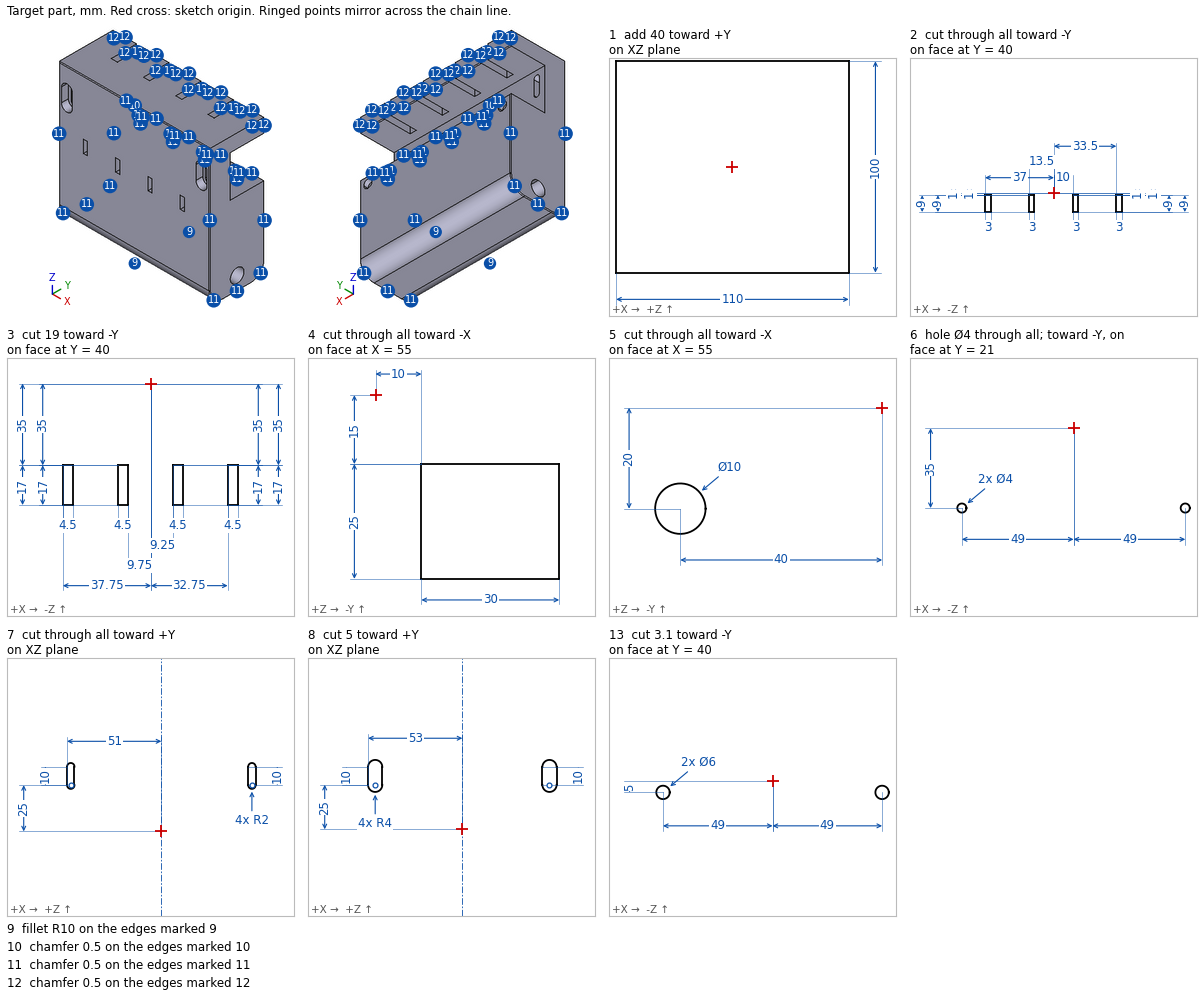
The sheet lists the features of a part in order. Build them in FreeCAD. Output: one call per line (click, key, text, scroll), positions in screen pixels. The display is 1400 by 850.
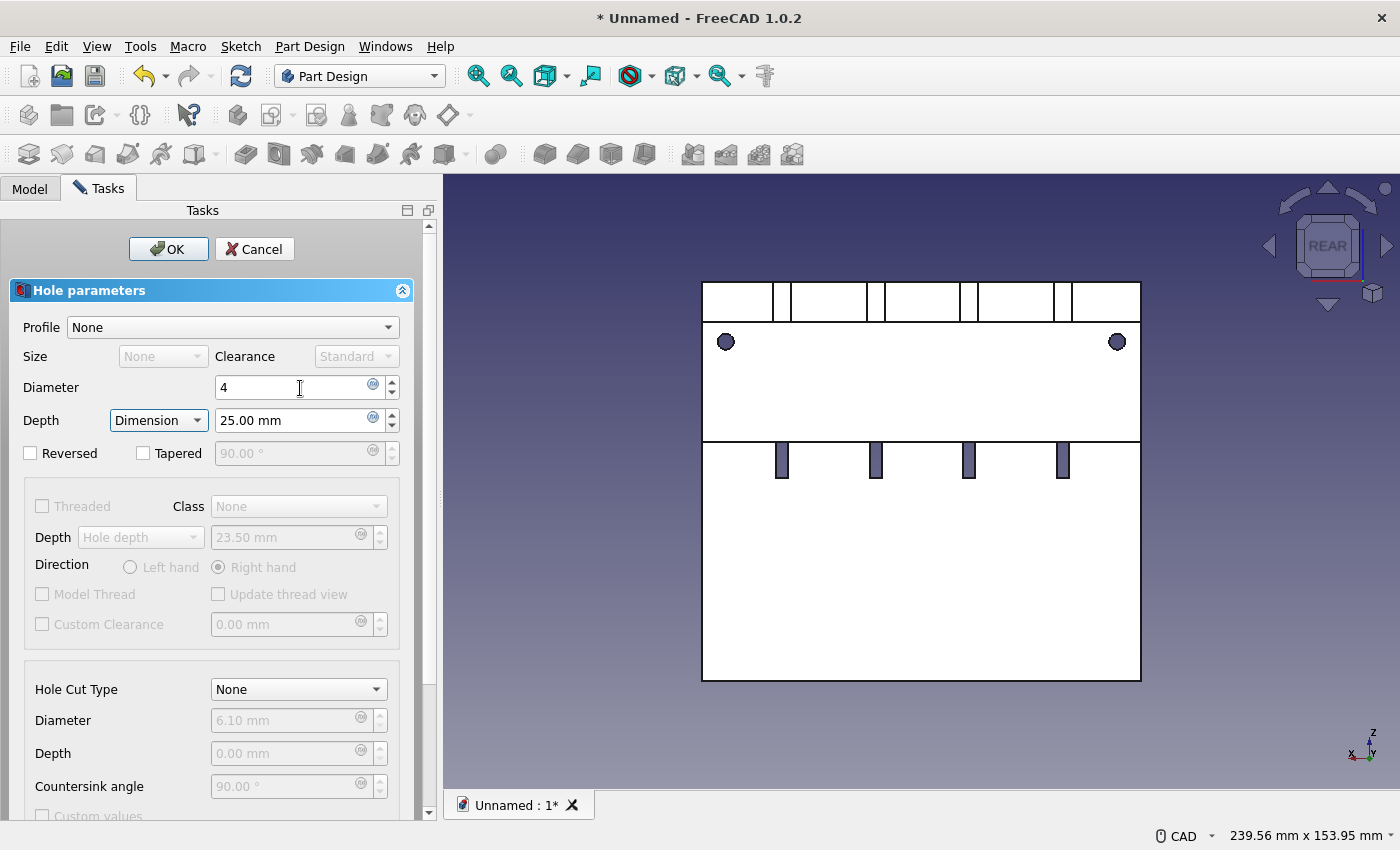
click(160, 420)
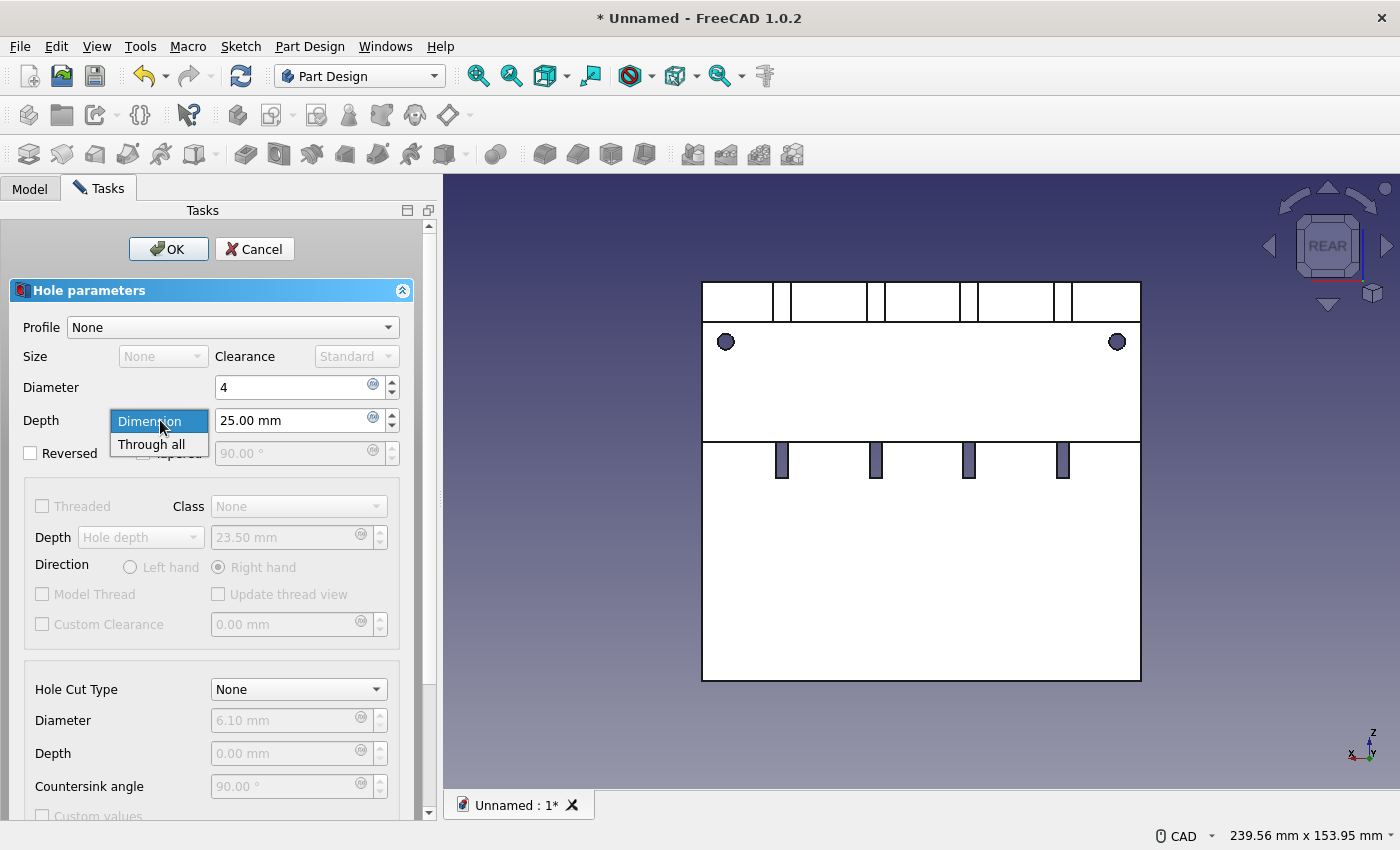
click(158, 444)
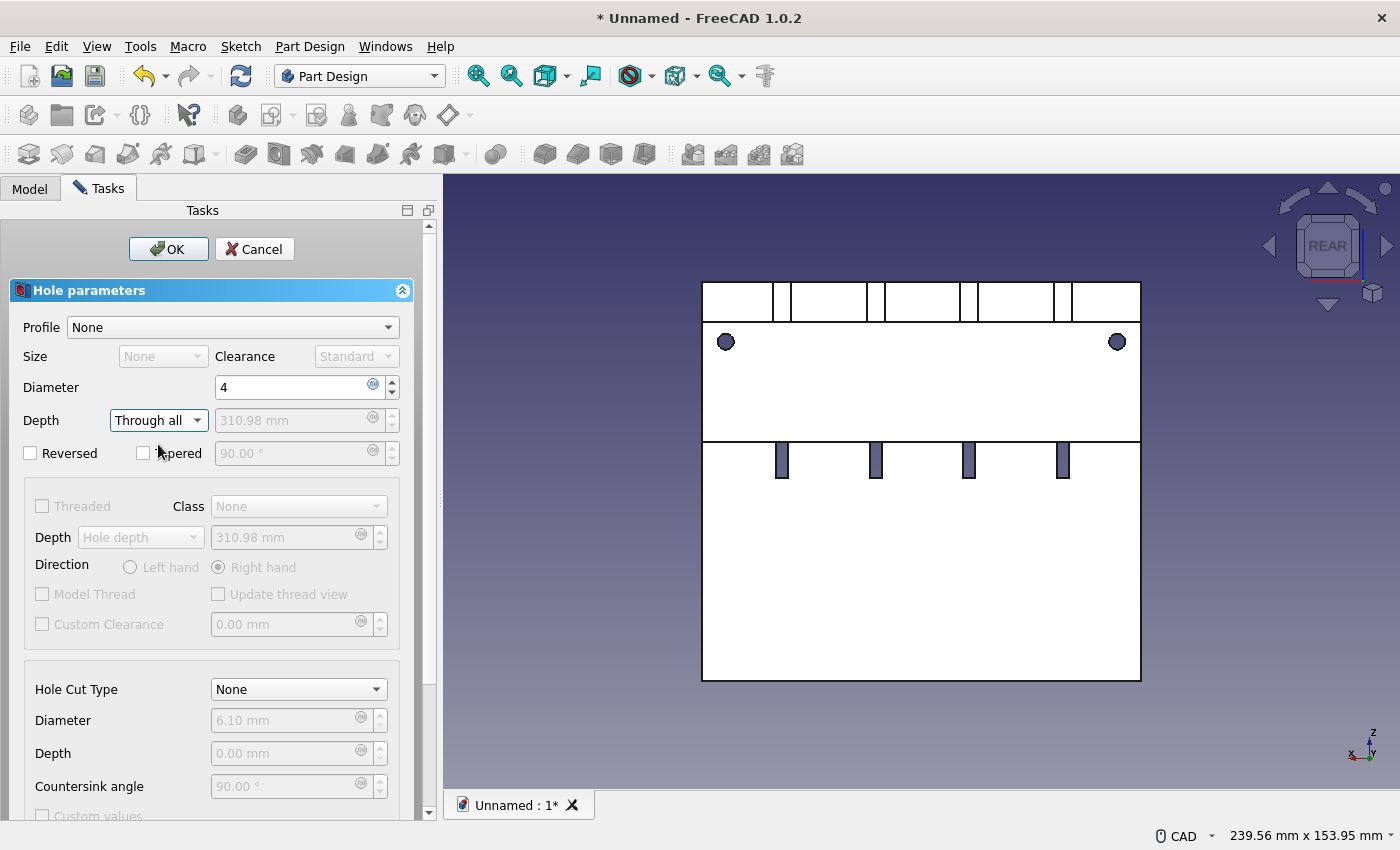
click(169, 249)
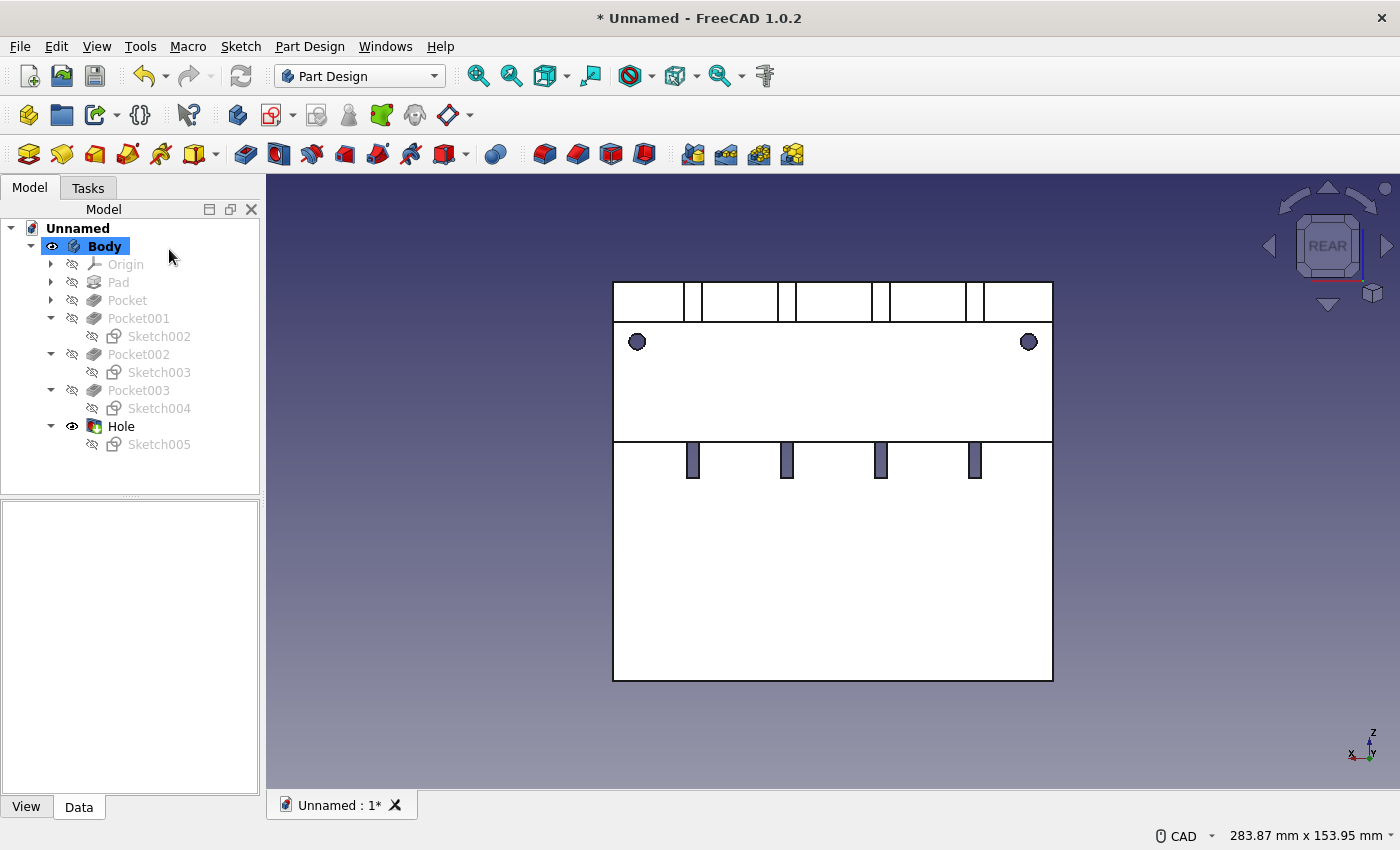
click(270, 116)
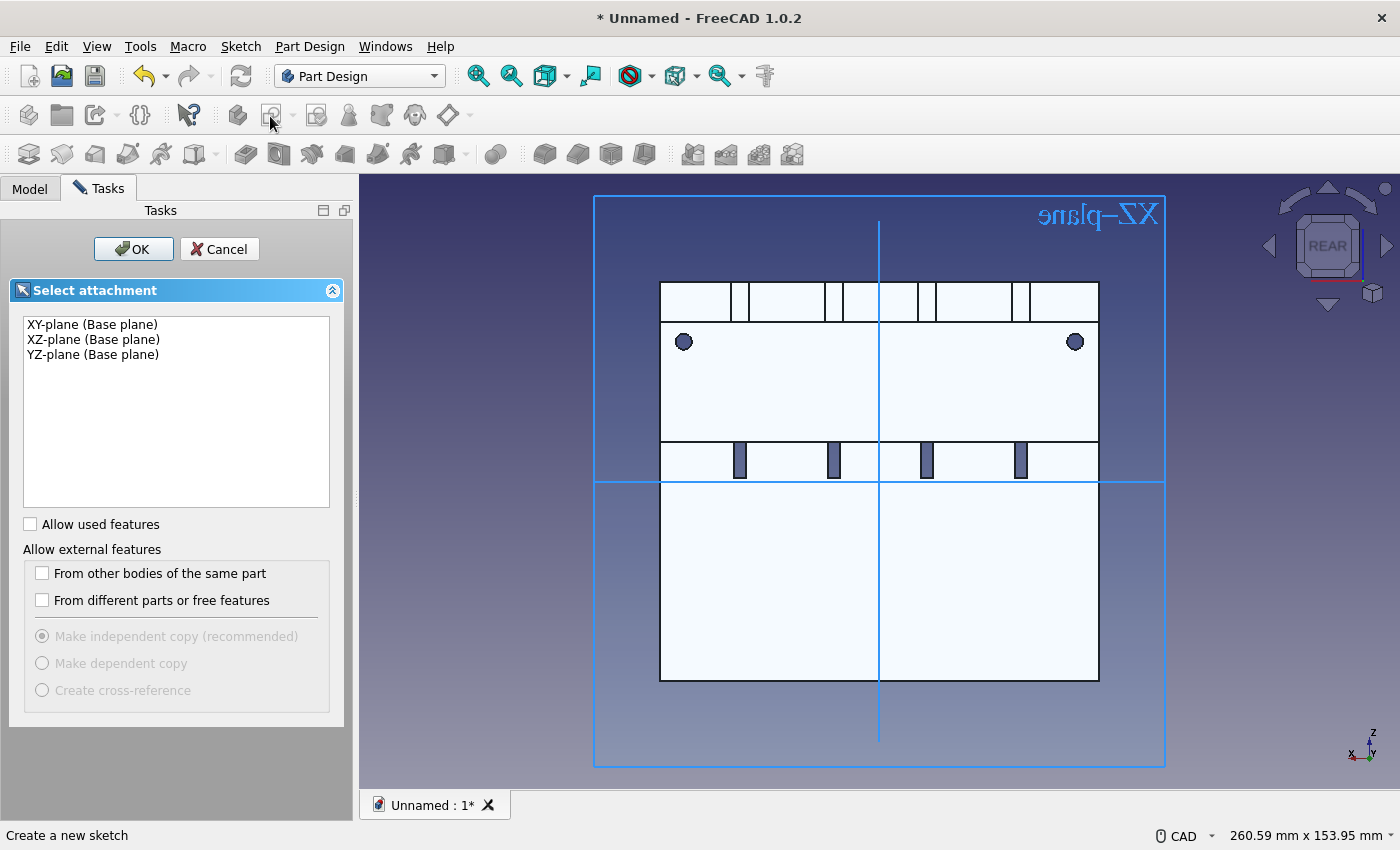
click(84, 340)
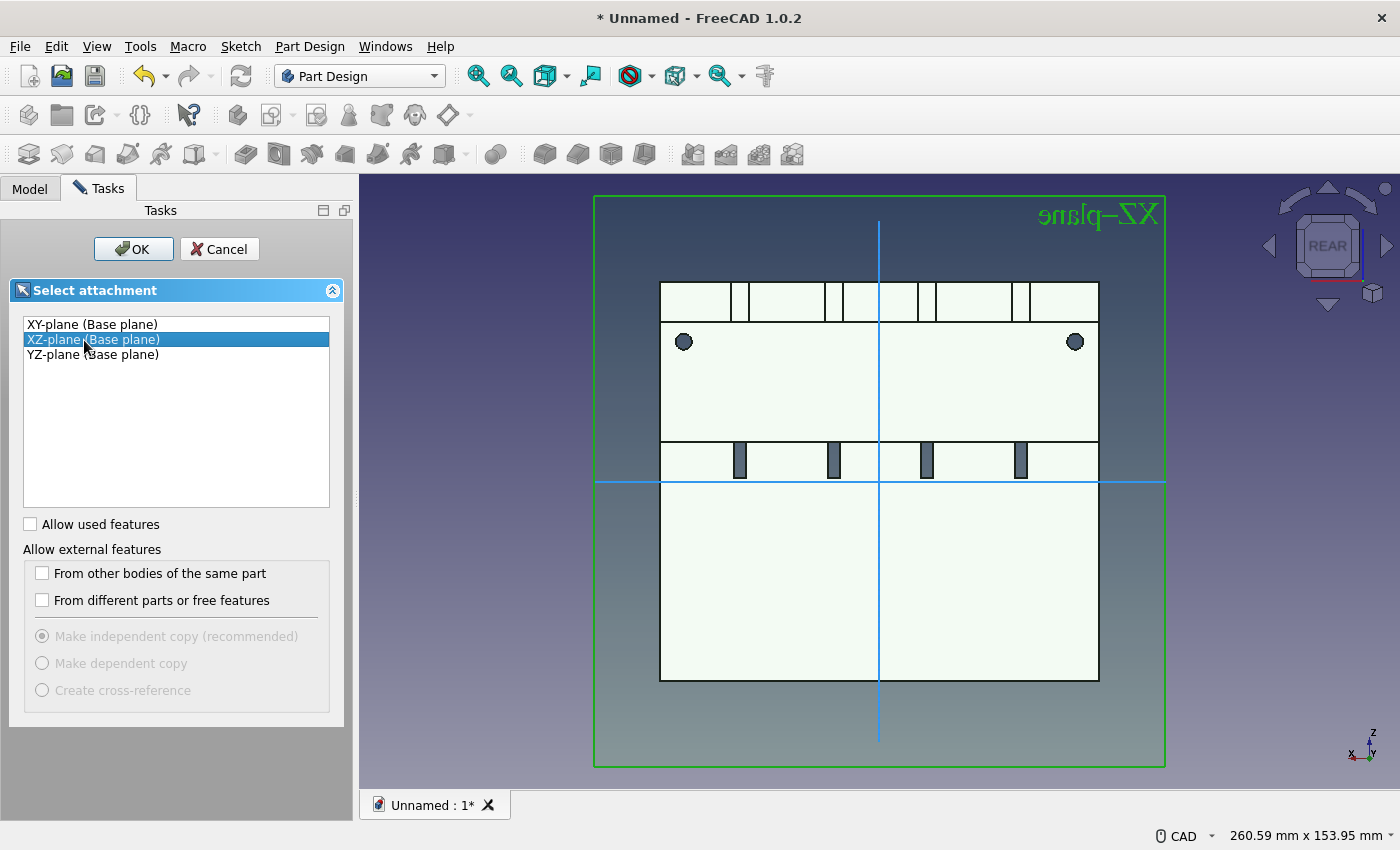
click(134, 249)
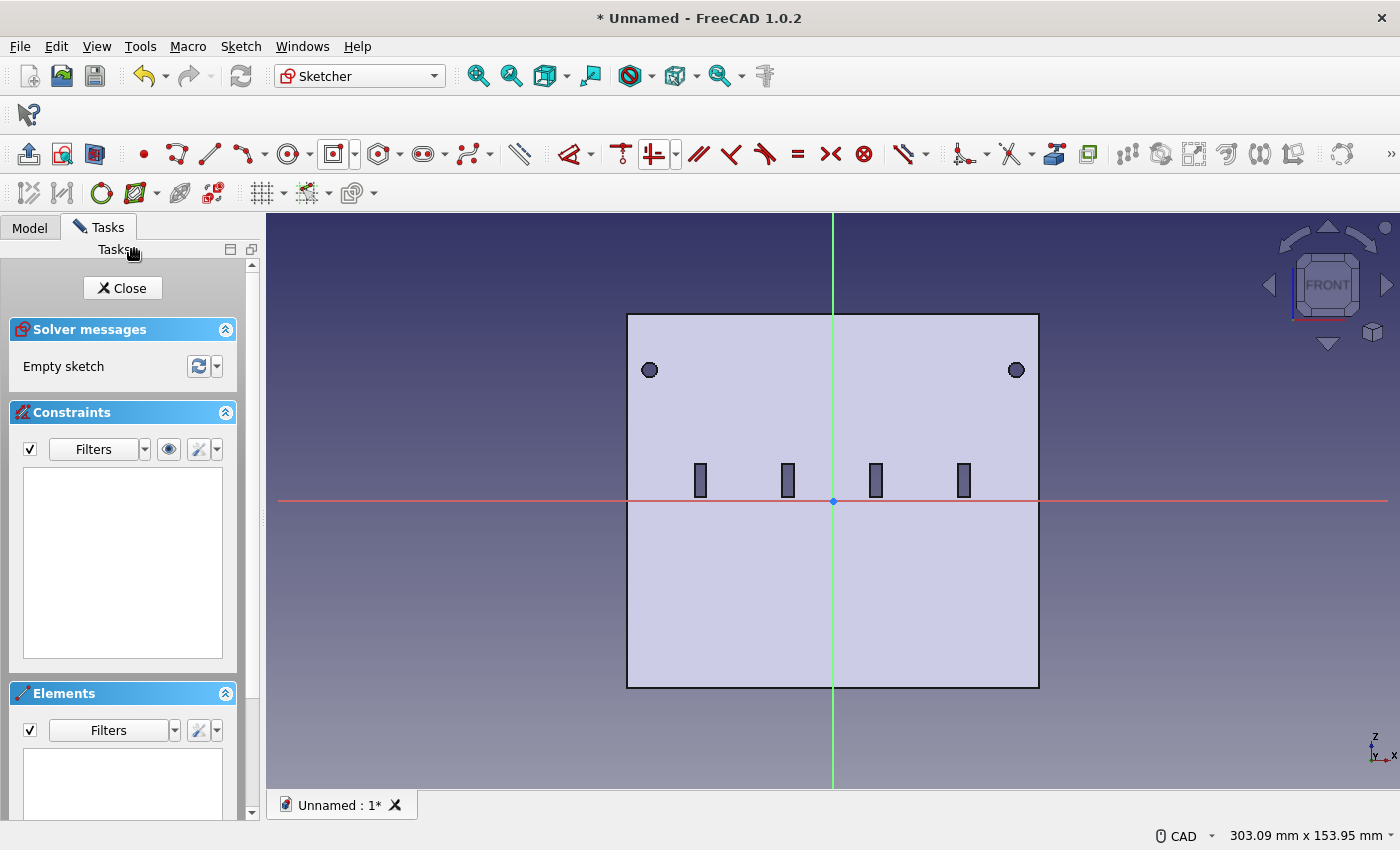
scroll(916, 348, up, 3)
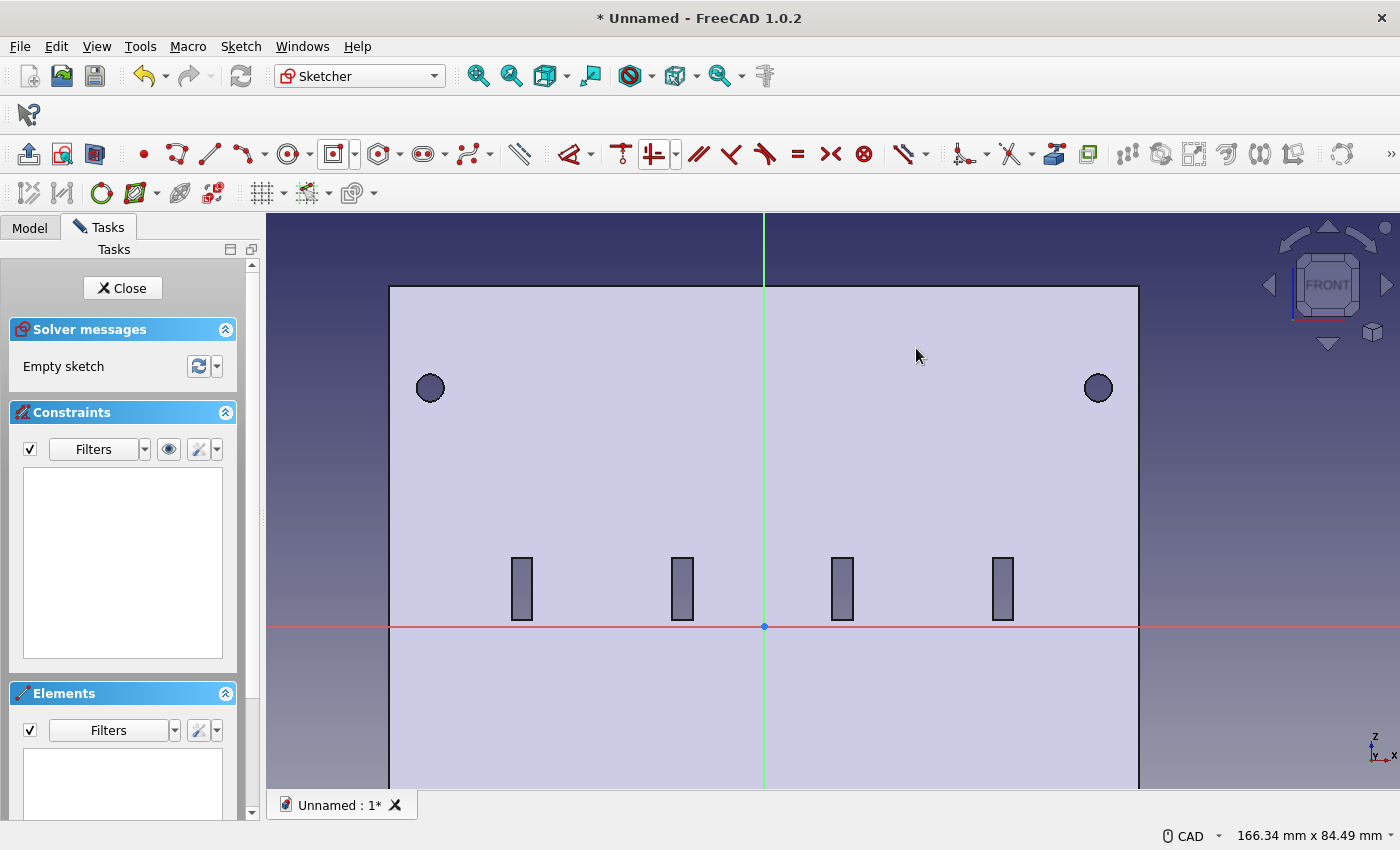
key(g)
key(s)